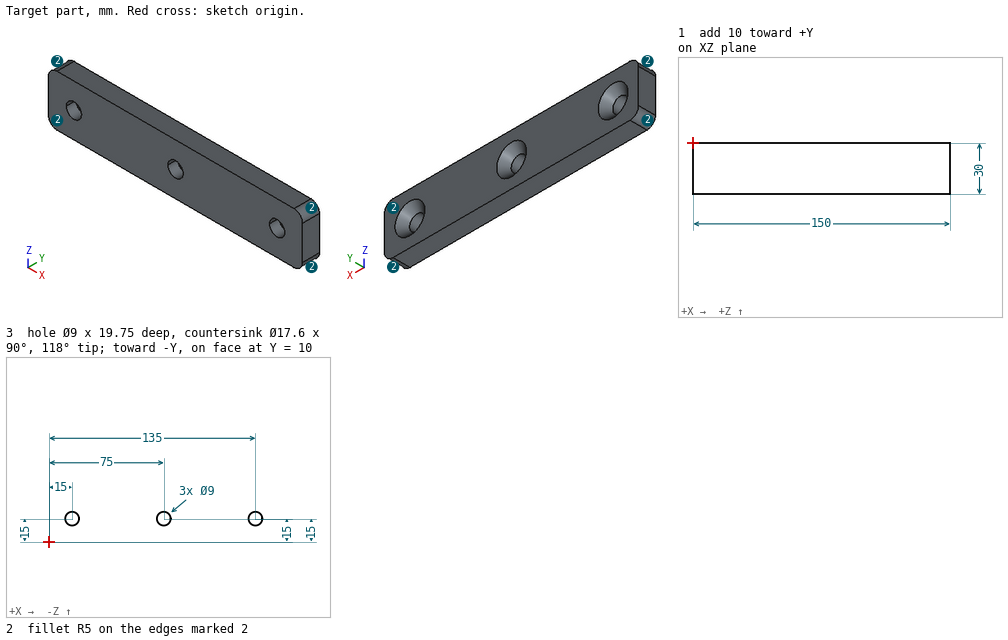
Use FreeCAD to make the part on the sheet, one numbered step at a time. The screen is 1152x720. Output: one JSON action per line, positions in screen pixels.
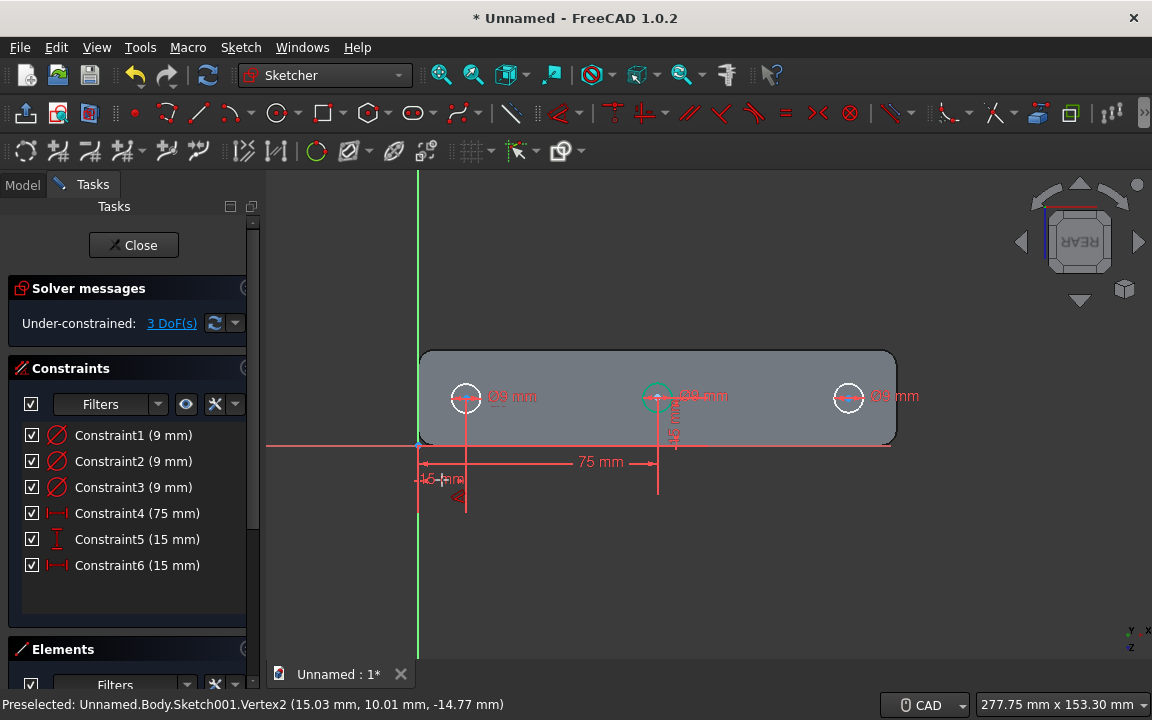
{"action": "left_click", "coordinate": [466, 398]}
{"action": "left_click", "coordinate": [384, 422]}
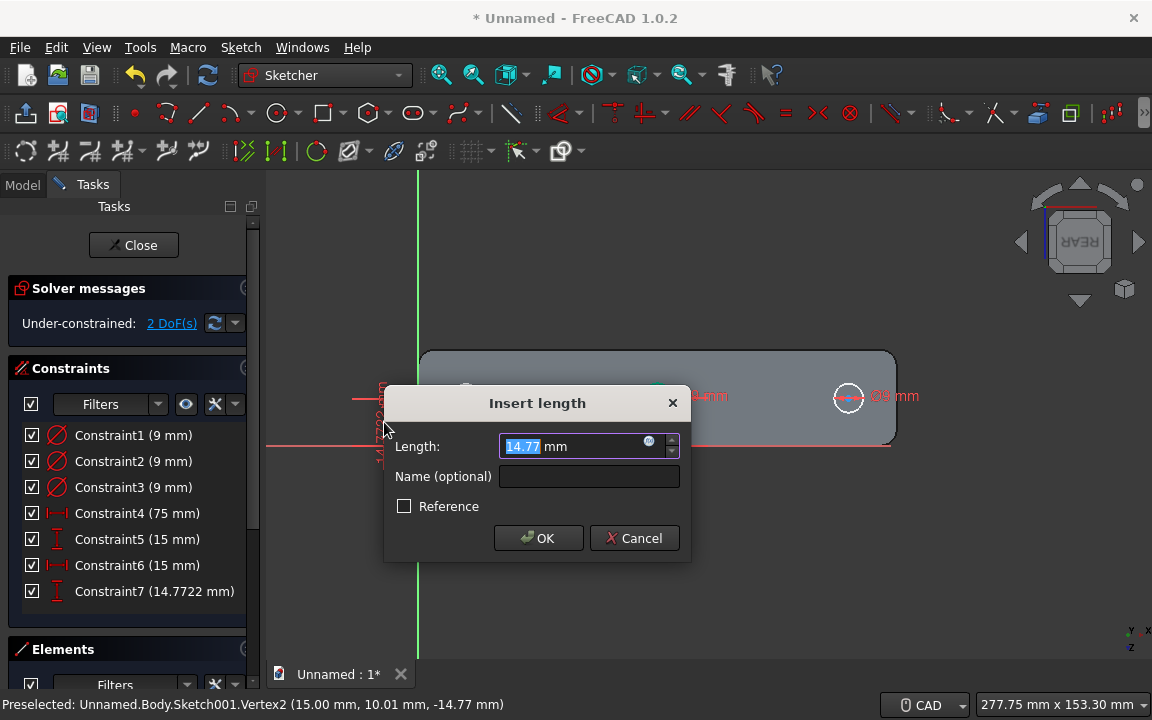
{"action": "type", "text": "15"}
{"action": "key", "text": "Return"}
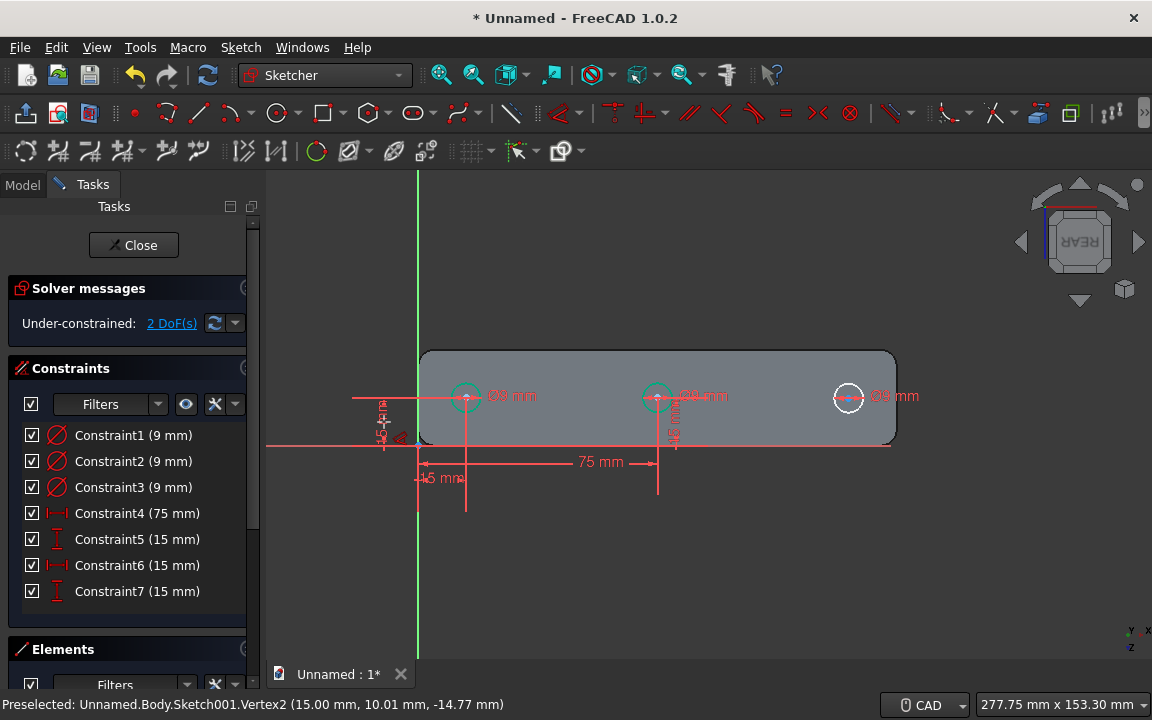
{"action": "left_click", "coordinate": [849, 398]}
{"action": "left_click", "coordinate": [883, 422]}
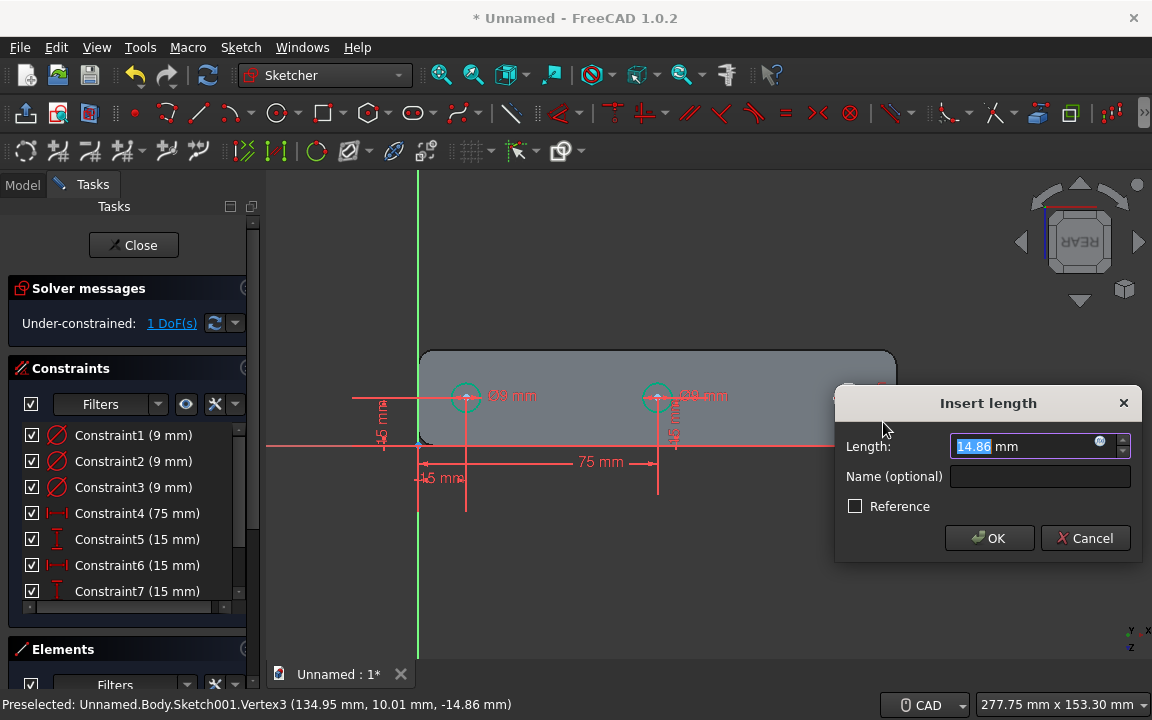
{"action": "type", "text": "15"}
{"action": "key", "text": "Return"}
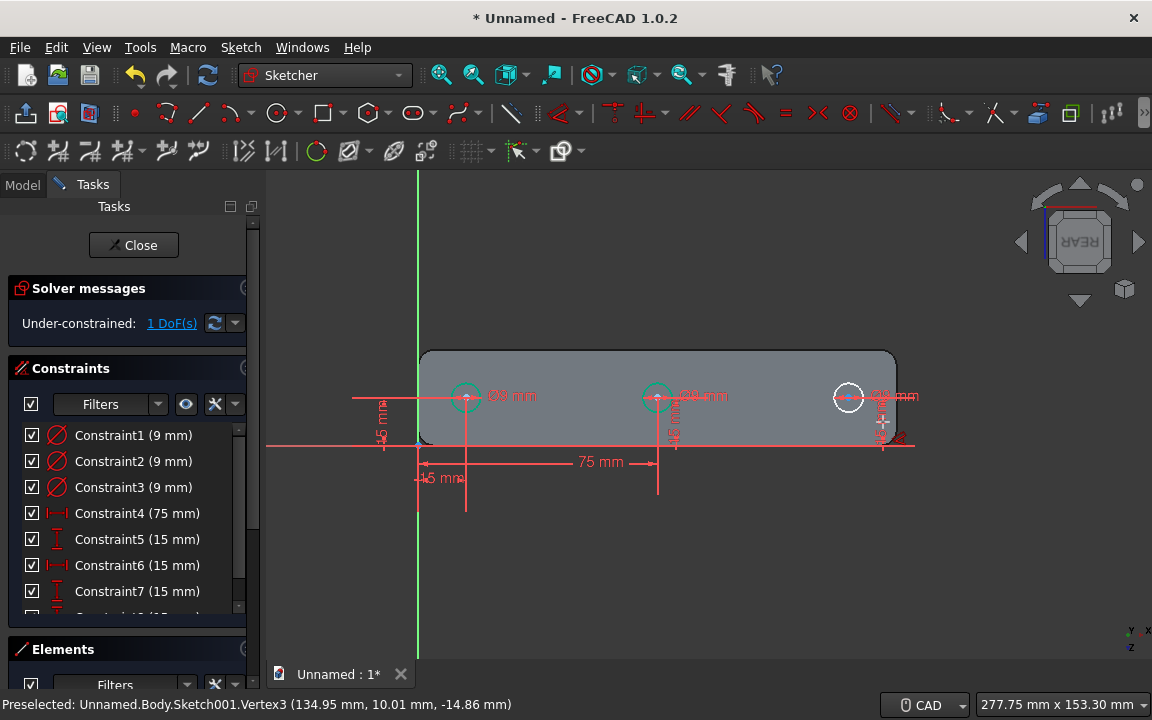
{"action": "left_click", "coordinate": [849, 398]}
{"action": "left_click", "coordinate": [733, 480]}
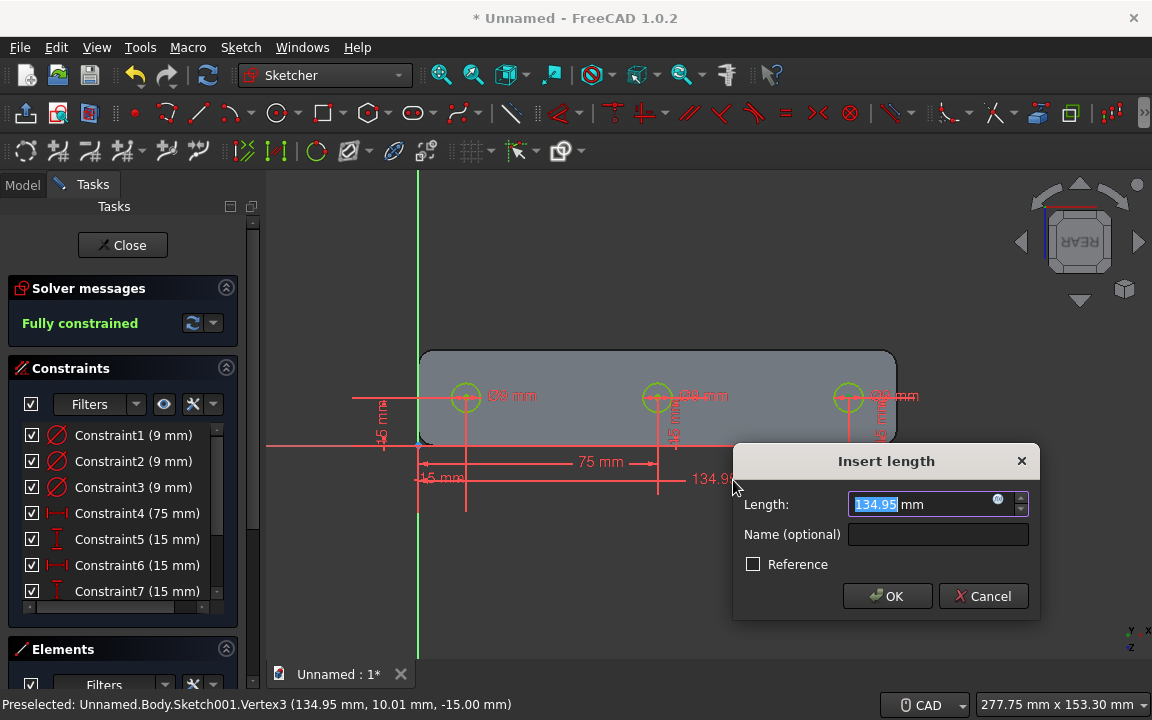
{"action": "type", "text": "135"}
{"action": "key", "text": "Return"}
{"action": "key", "text": "Escape"}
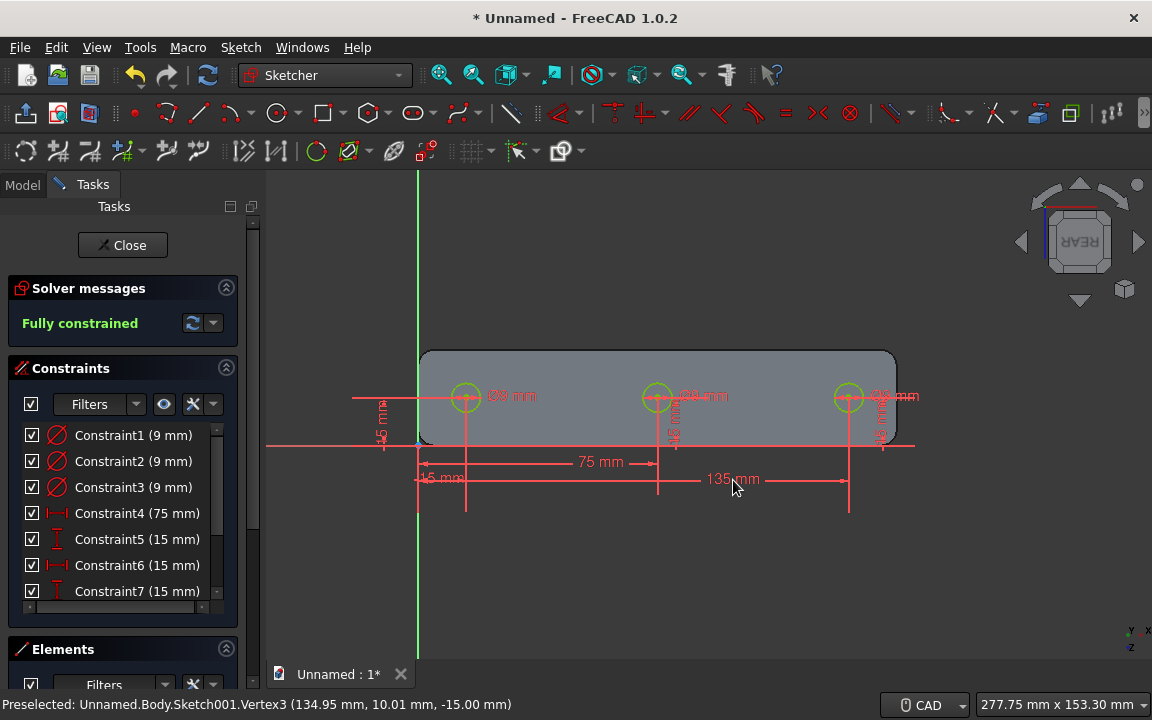
{"action": "left_click", "coordinate": [123, 245]}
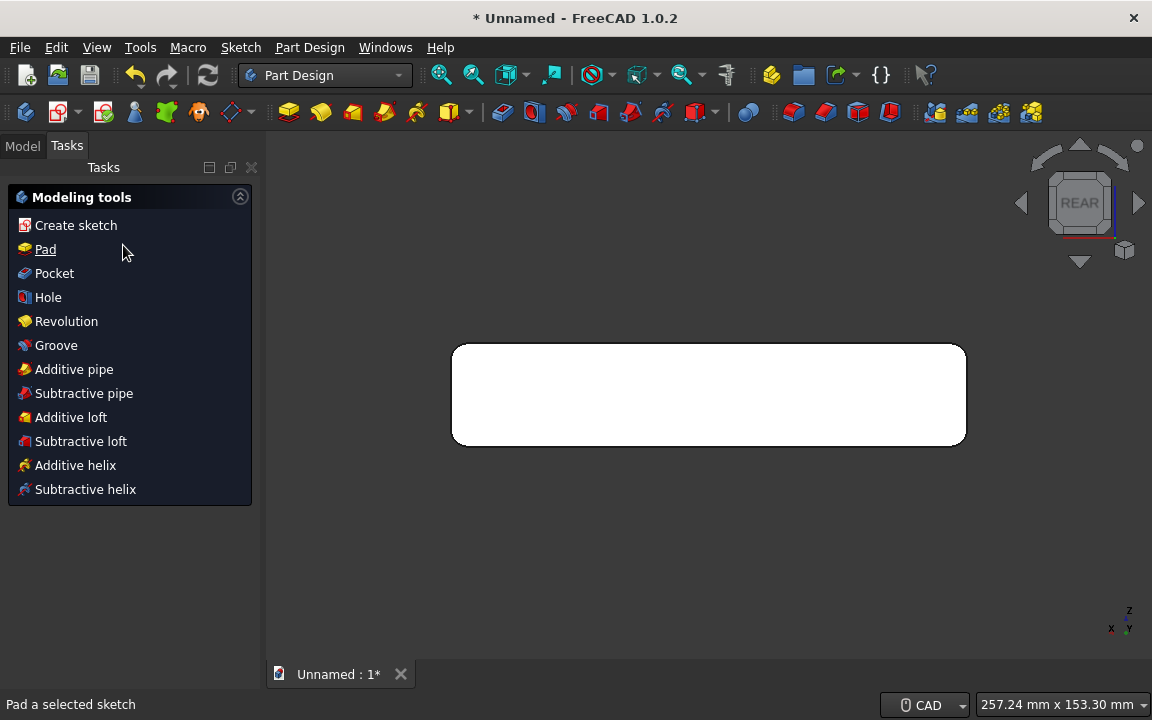
{"action": "left_click", "coordinate": [536, 112]}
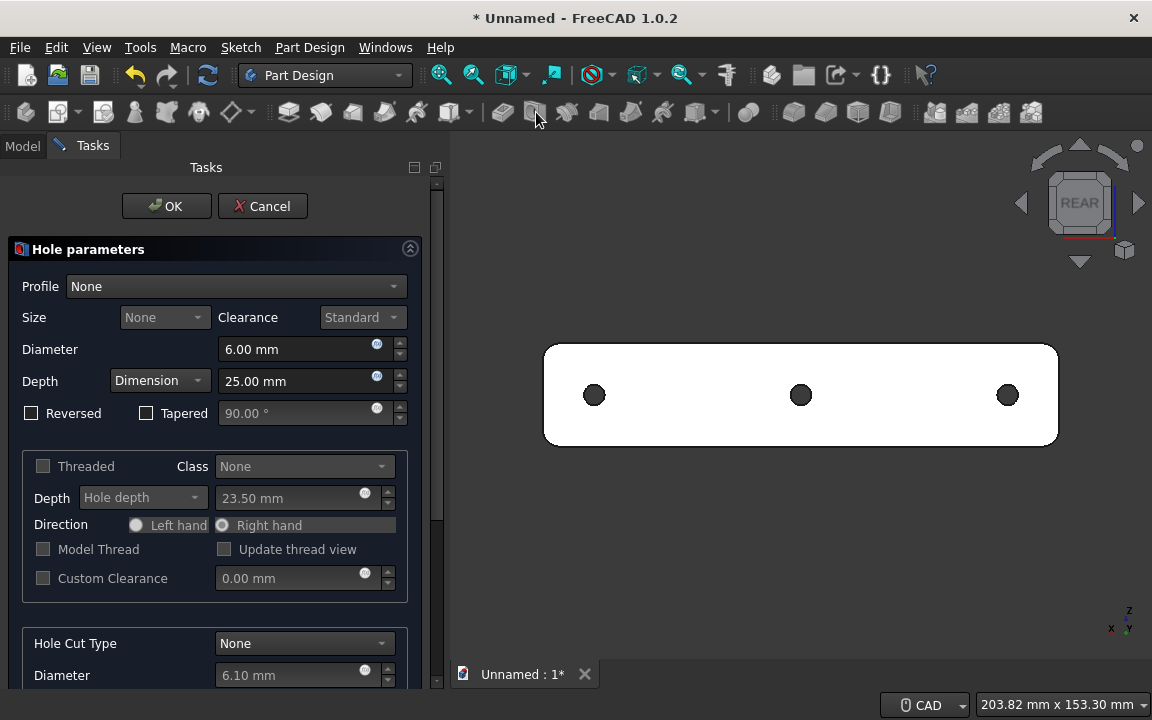
{"action": "triple_click", "coordinate": [305, 349]}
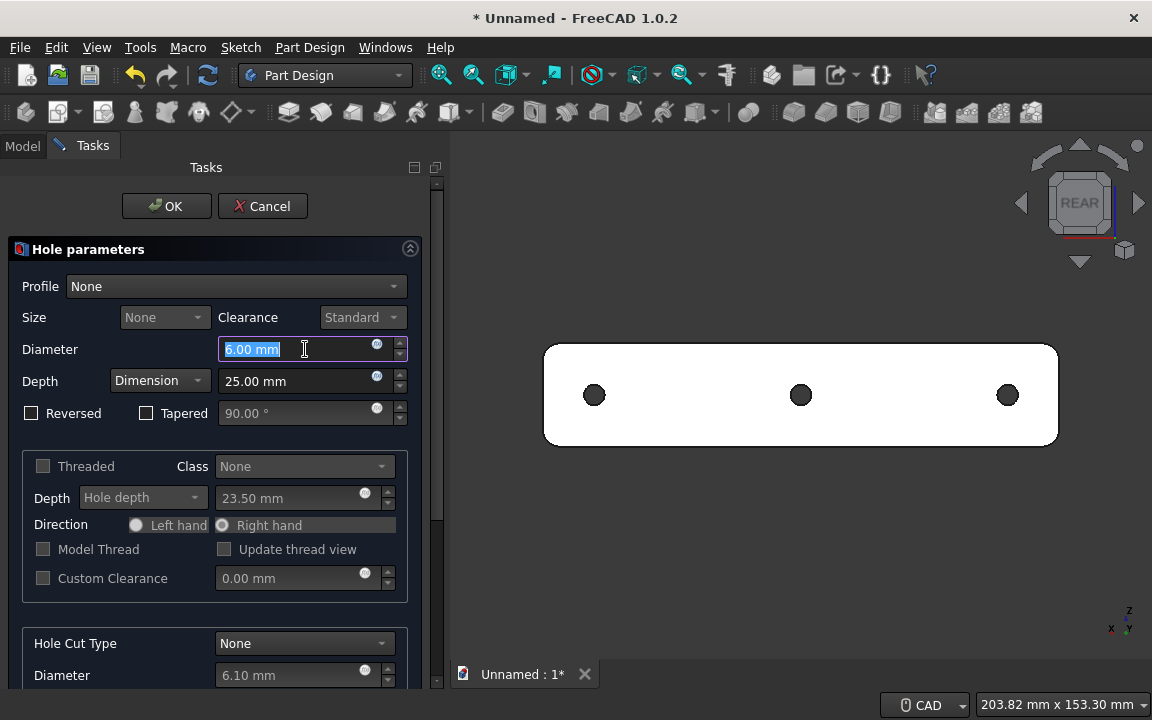
{"action": "type", "text": "9"}
{"action": "key", "text": "Tab"}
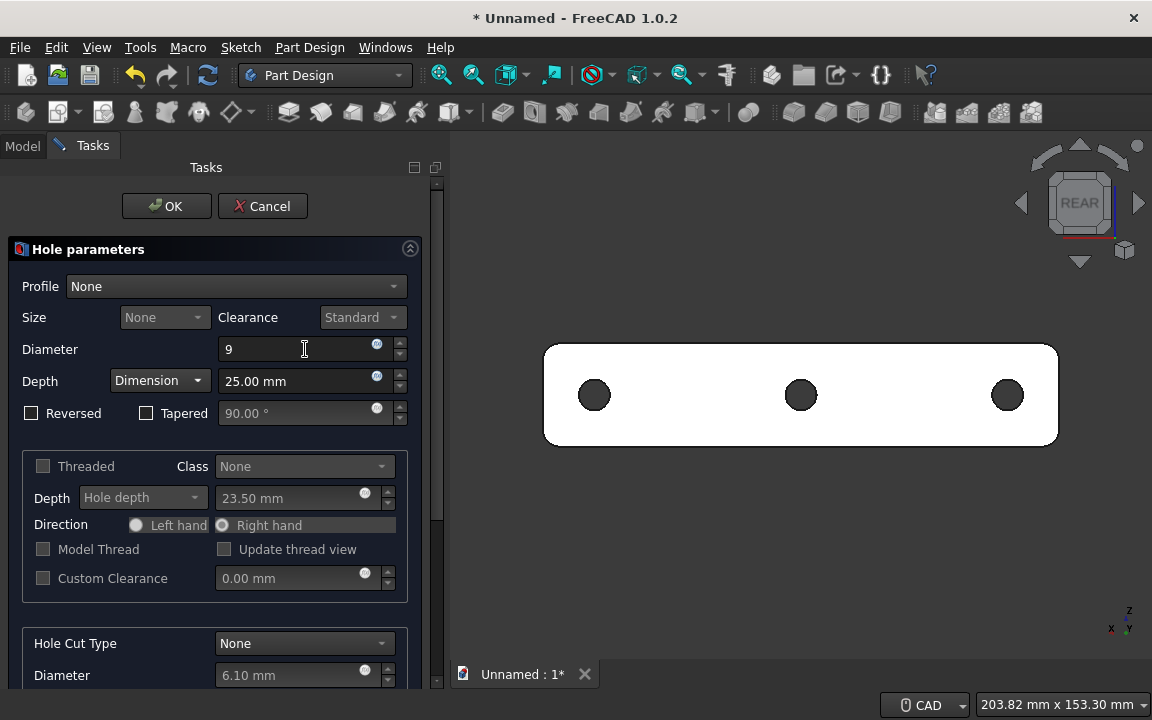
{"action": "triple_click", "coordinate": [305, 381]}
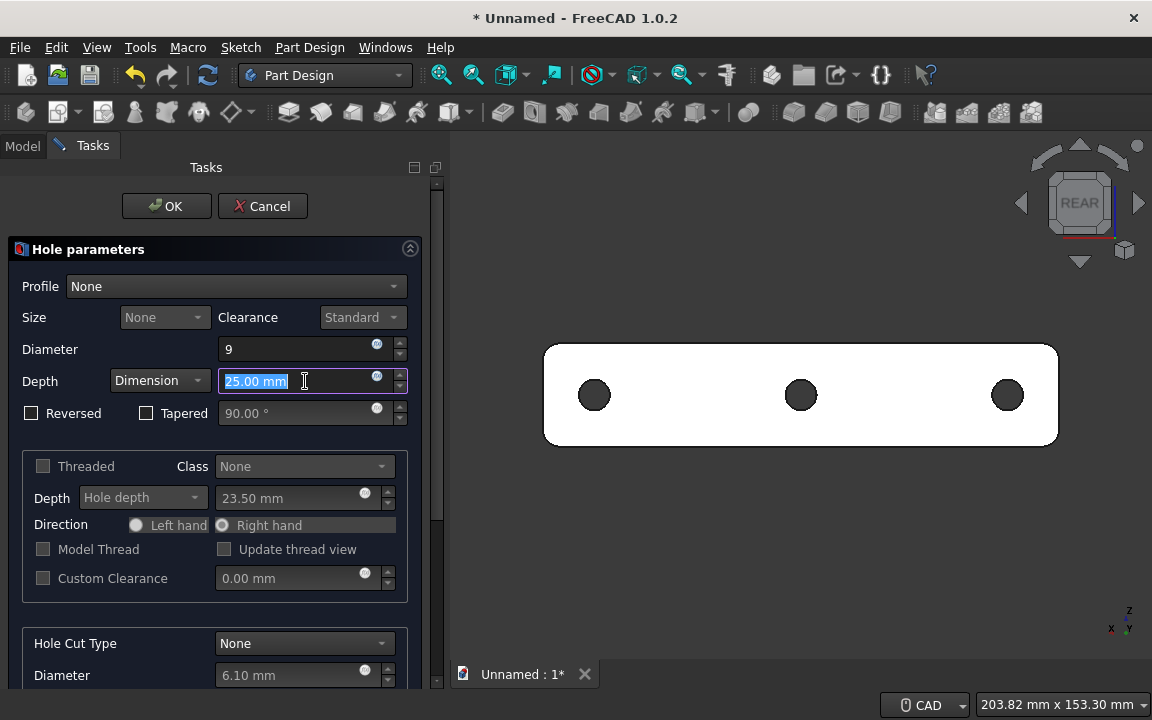
{"action": "type", "text": "19.75"}
{"action": "key", "text": "Tab"}